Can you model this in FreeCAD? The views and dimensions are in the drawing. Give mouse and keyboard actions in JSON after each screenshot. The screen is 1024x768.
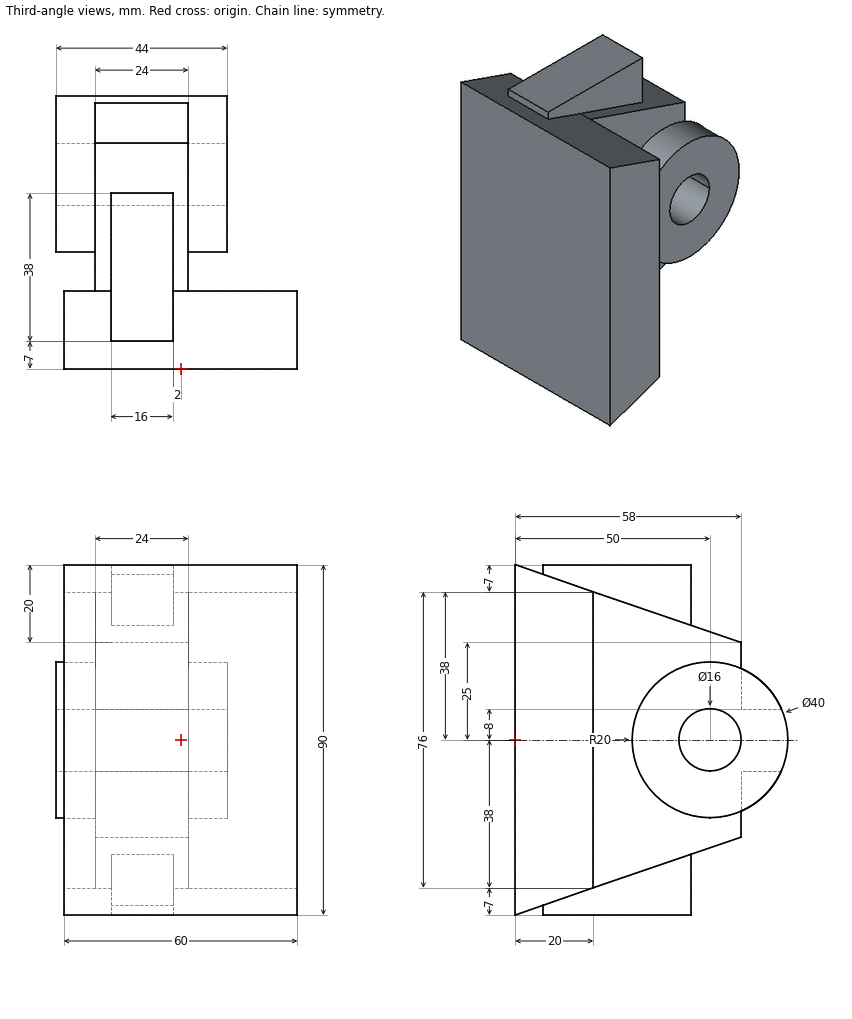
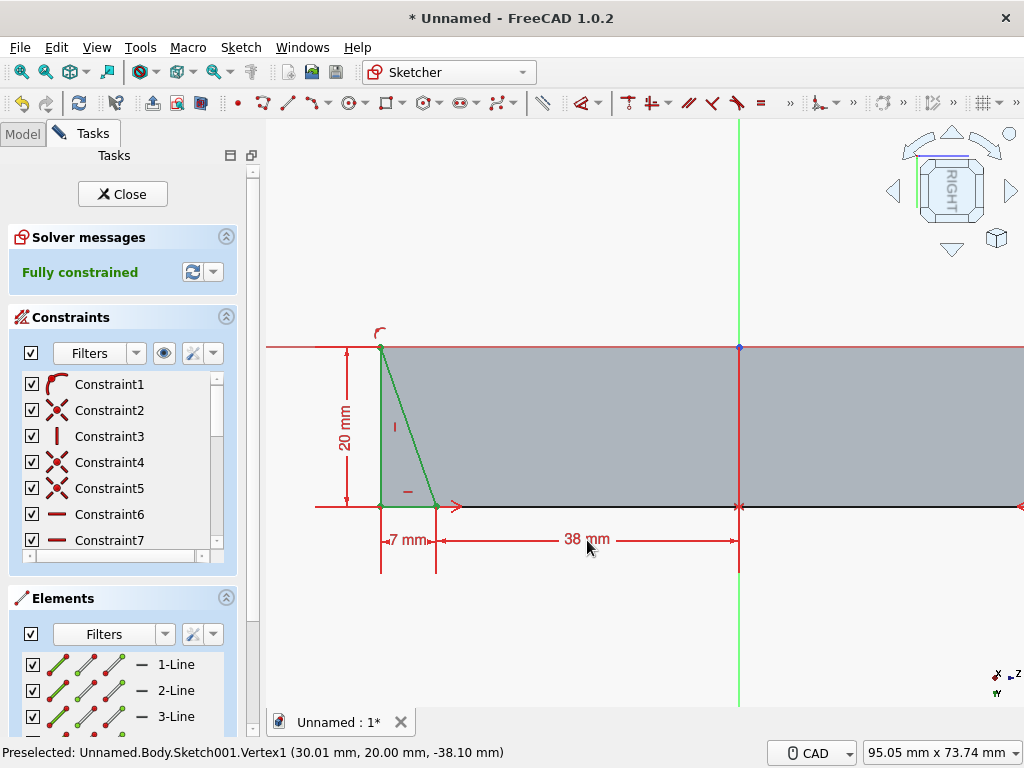
{"action": "left_click", "coordinate": [123, 194]}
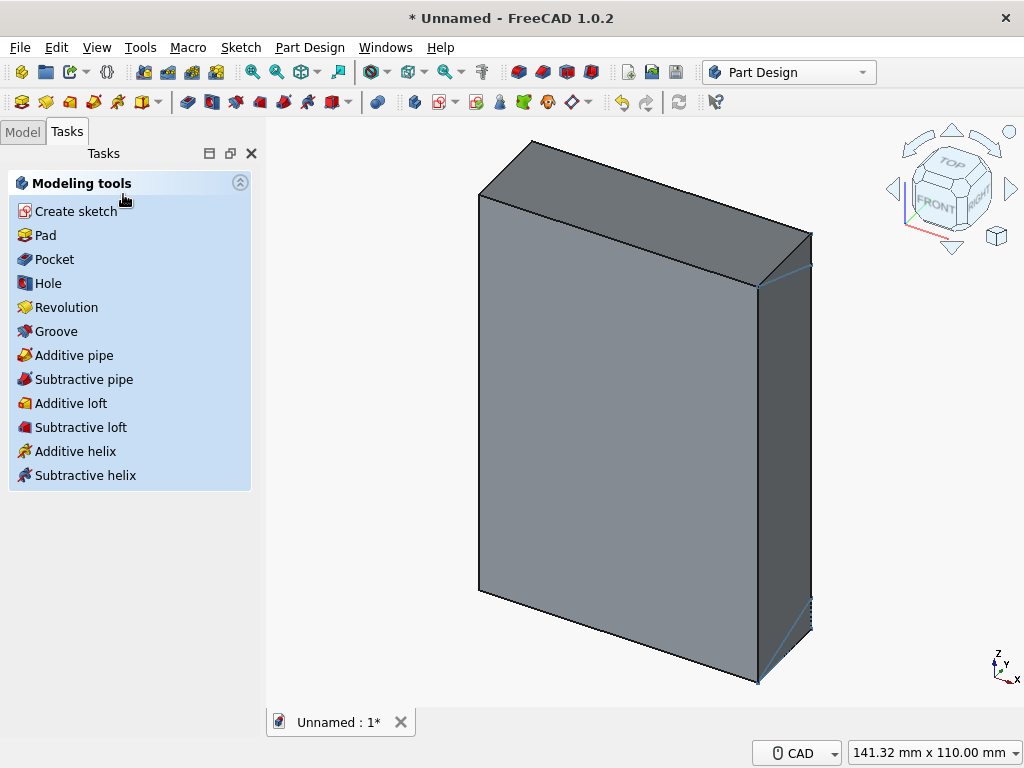
{"action": "left_click", "coordinate": [188, 102]}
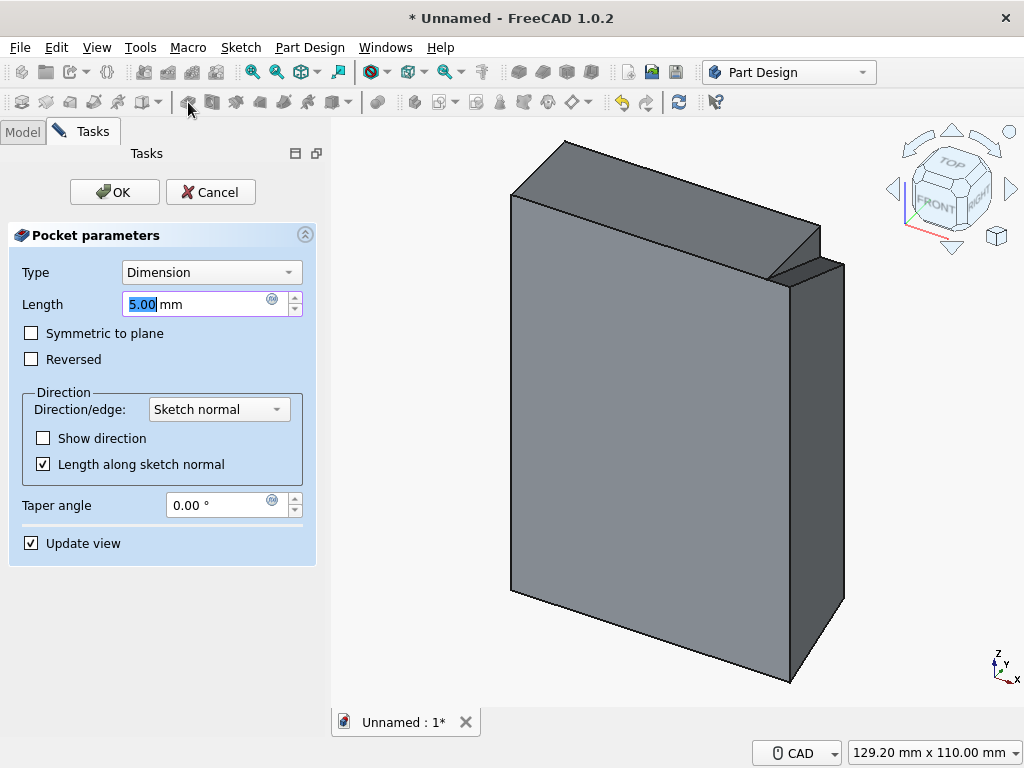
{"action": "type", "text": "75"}
{"action": "key", "text": "Tab"}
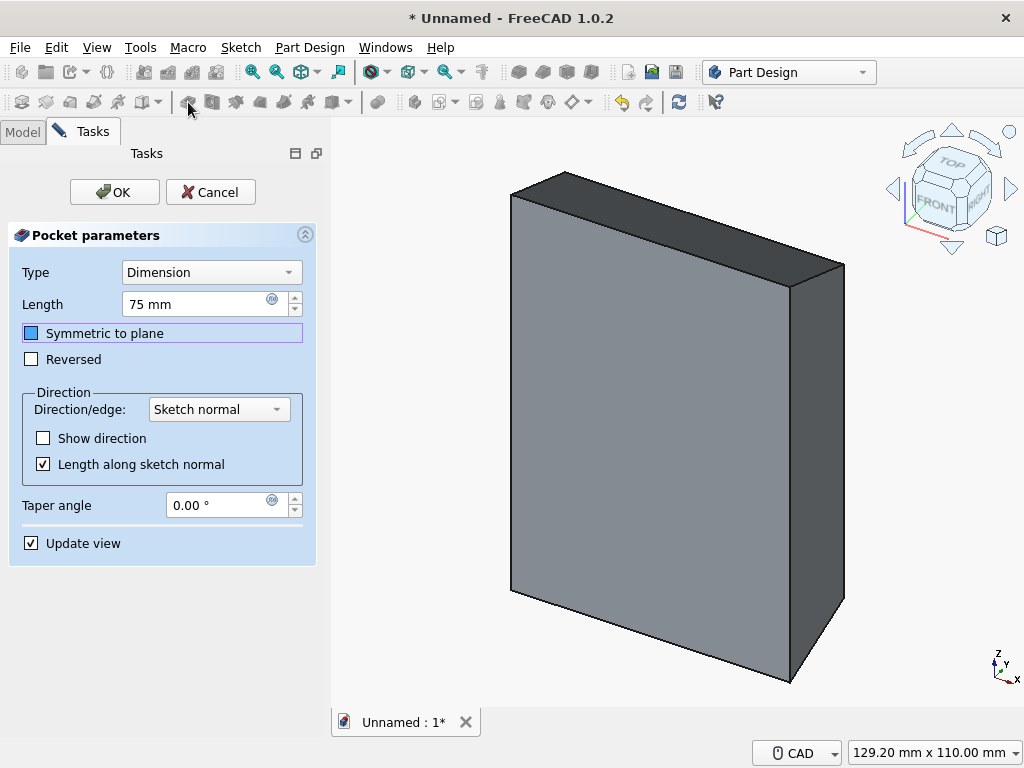
{"action": "left_click", "coordinate": [115, 192]}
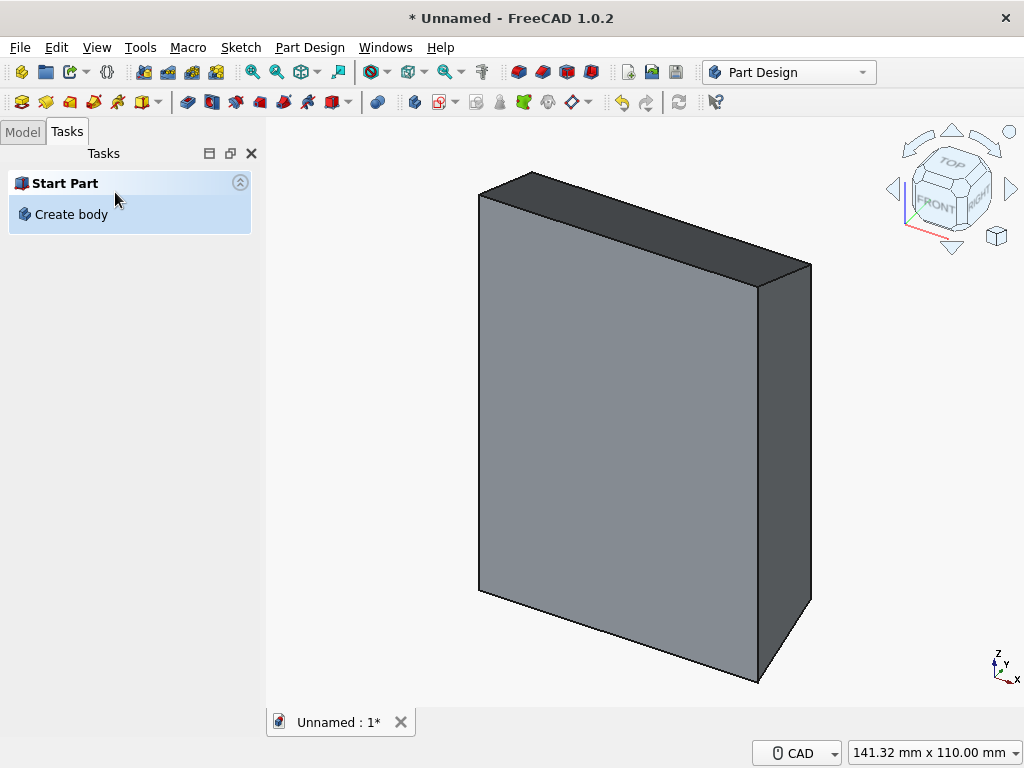
{"action": "left_click", "coordinate": [416, 102]}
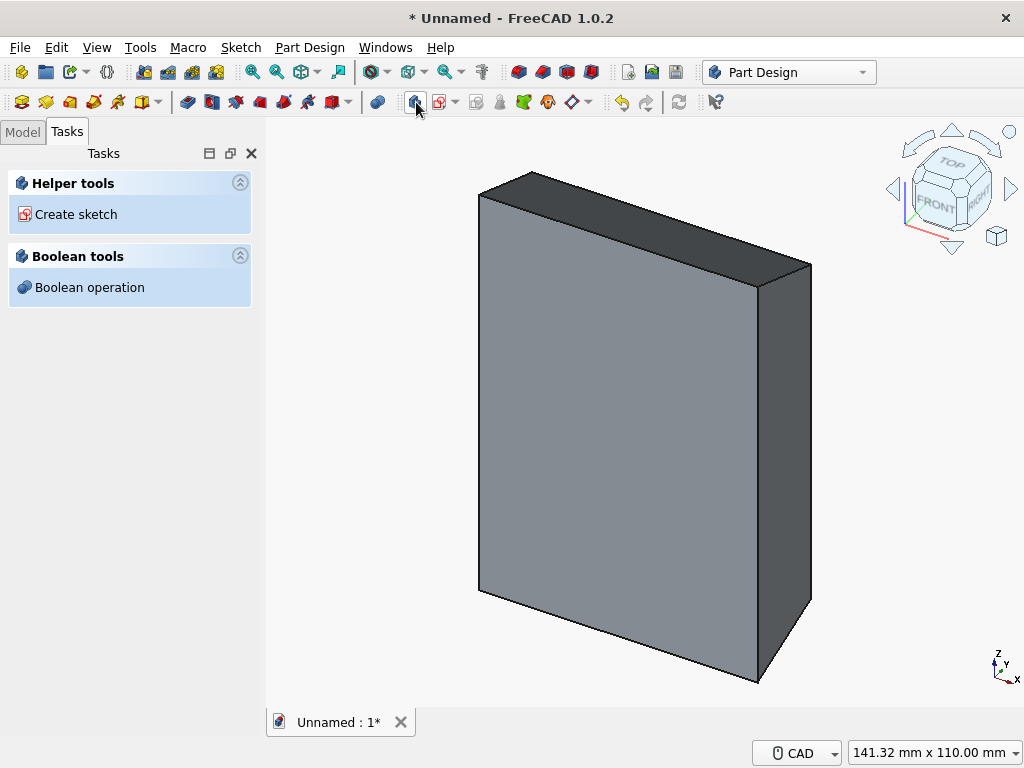
{"action": "left_click", "coordinate": [23, 131]}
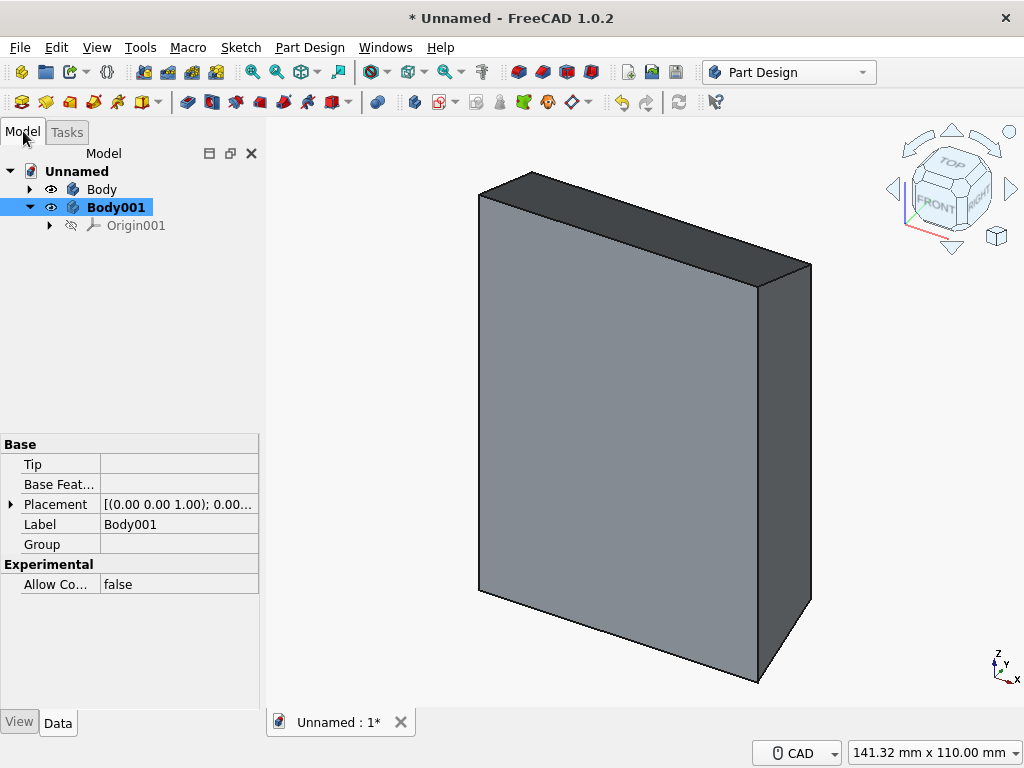
{"action": "left_click", "coordinate": [50, 225]}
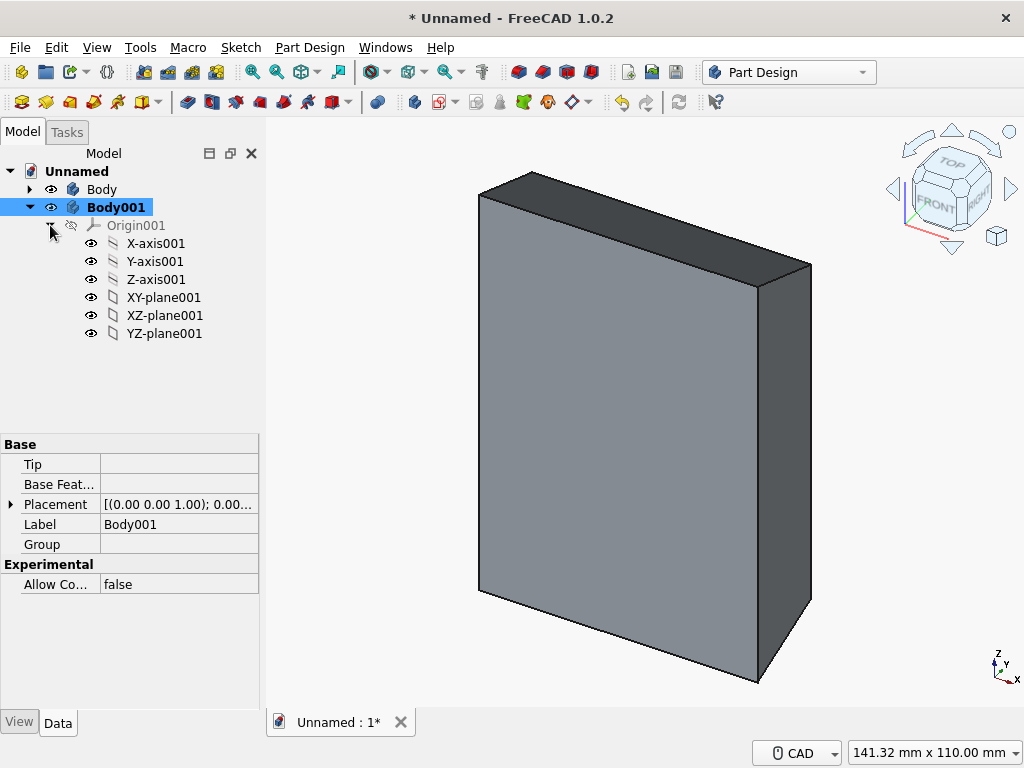
{"action": "left_click", "coordinate": [136, 333]}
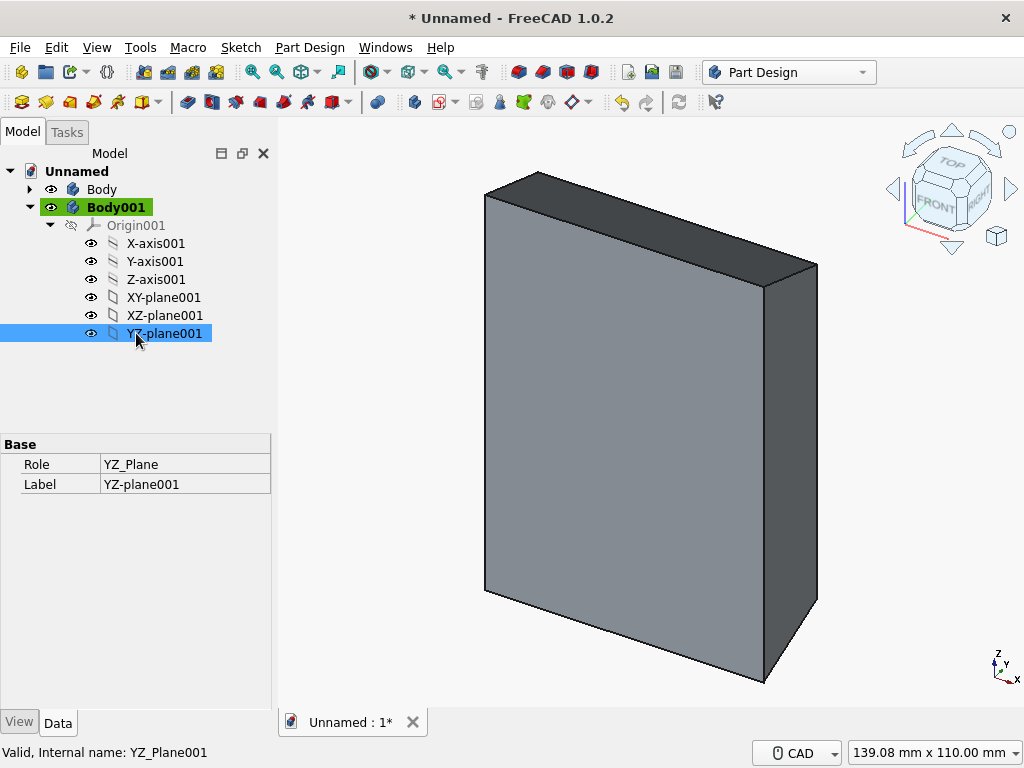
{"action": "left_click", "coordinate": [572, 102]}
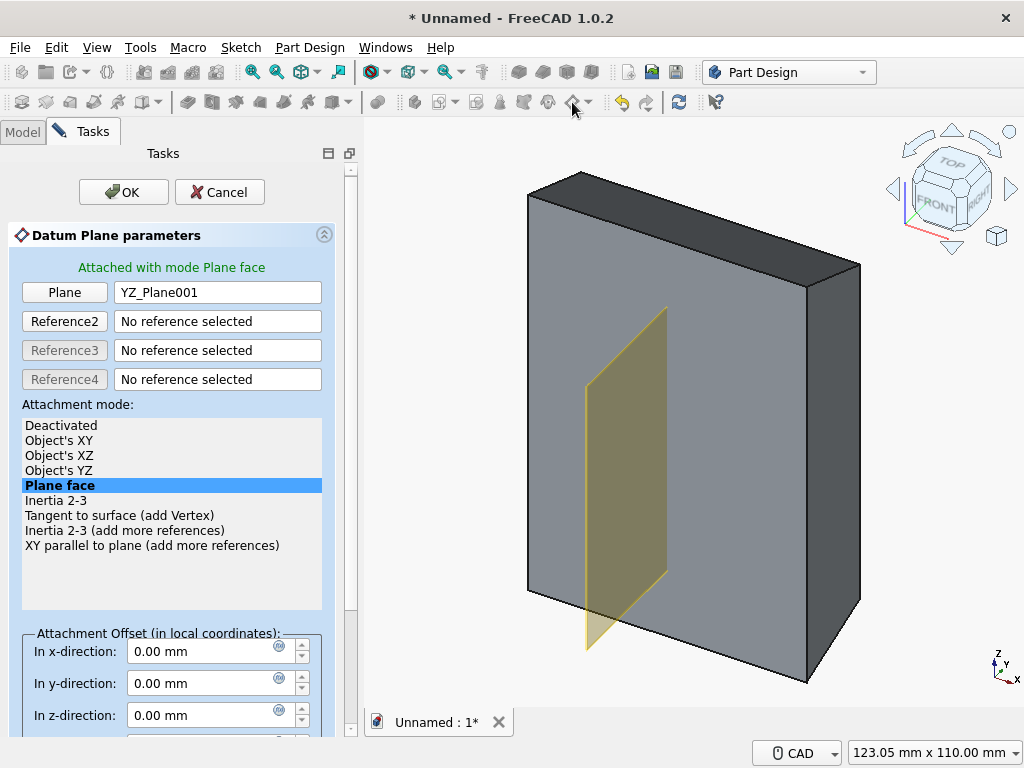
{"action": "triple_click", "coordinate": [210, 715]}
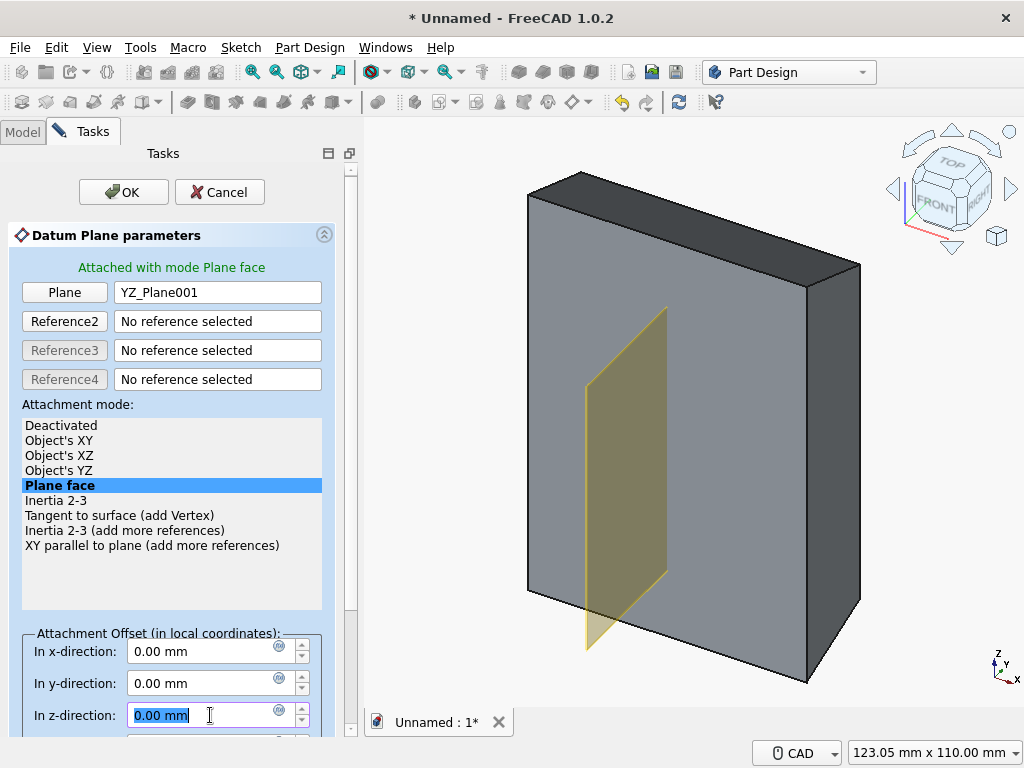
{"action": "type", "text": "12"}
{"action": "key", "text": "Tab"}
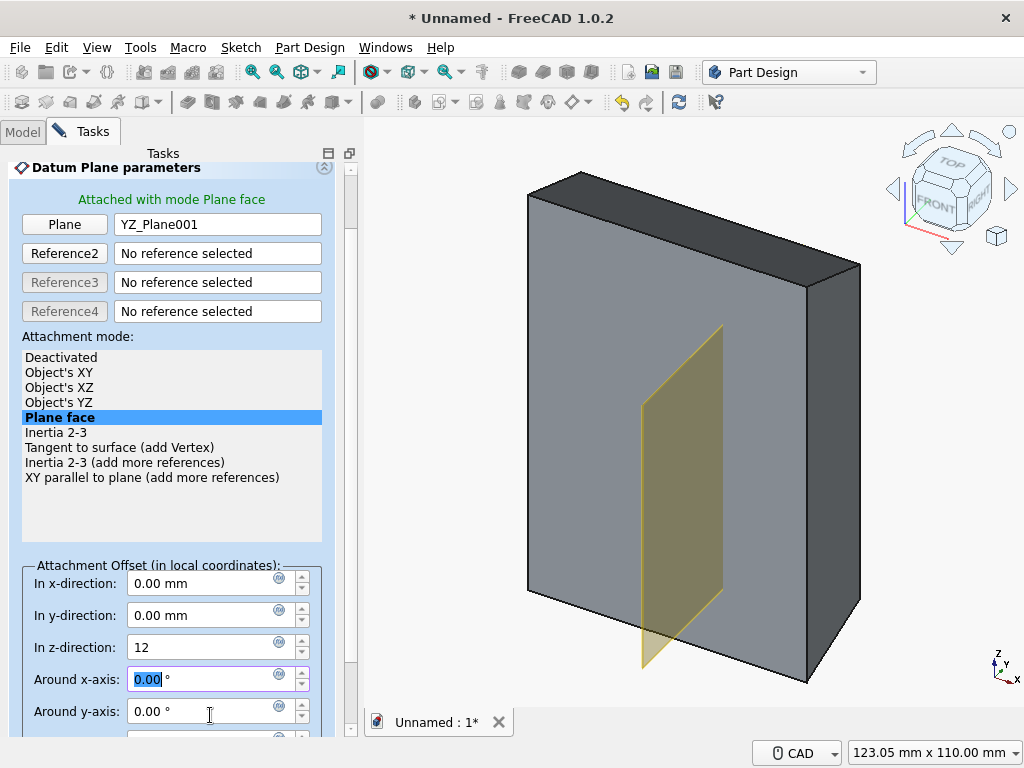
{"action": "scroll", "coordinate": [351, 450], "scroll_direction": "up", "scroll_amount": 2}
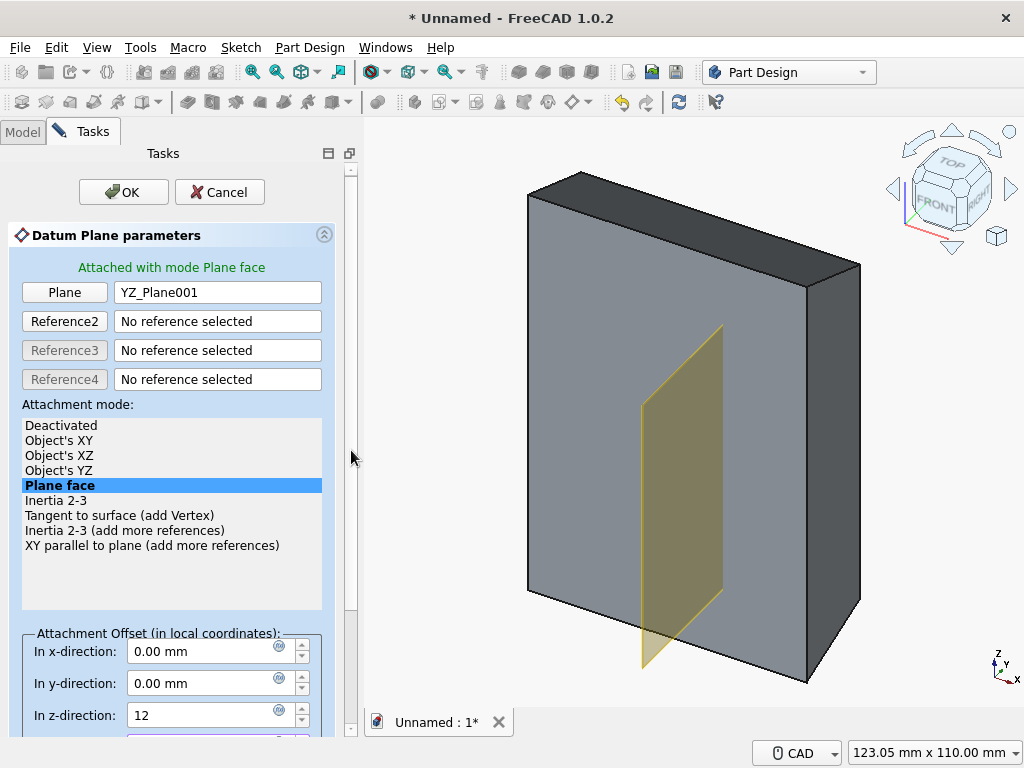
{"action": "left_click", "coordinate": [124, 192]}